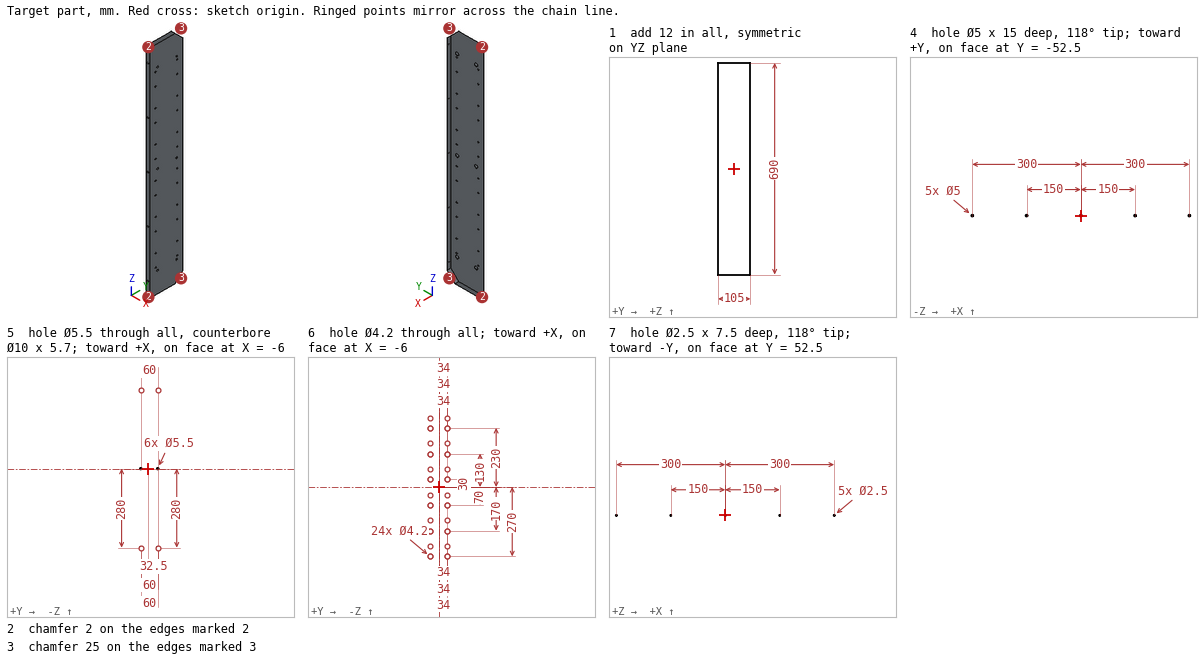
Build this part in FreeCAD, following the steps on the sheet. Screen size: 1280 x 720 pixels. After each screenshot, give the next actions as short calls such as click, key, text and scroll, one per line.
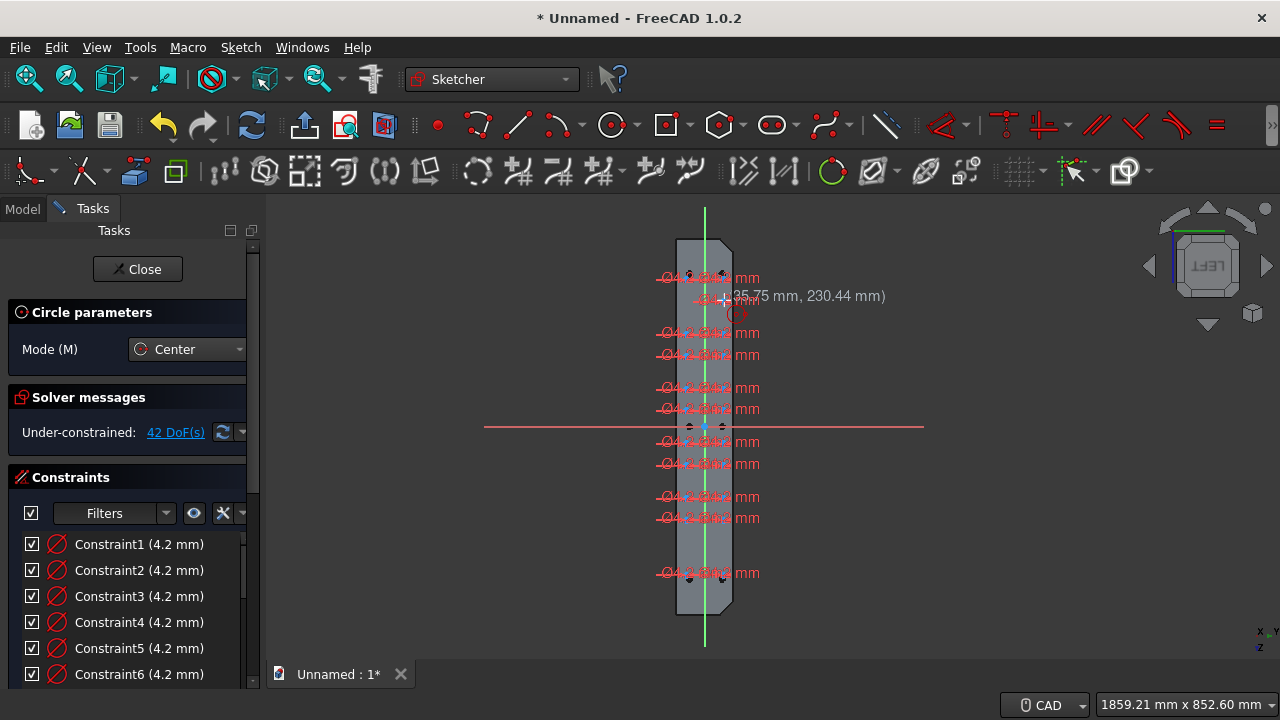
scroll(686, 301, up, 15)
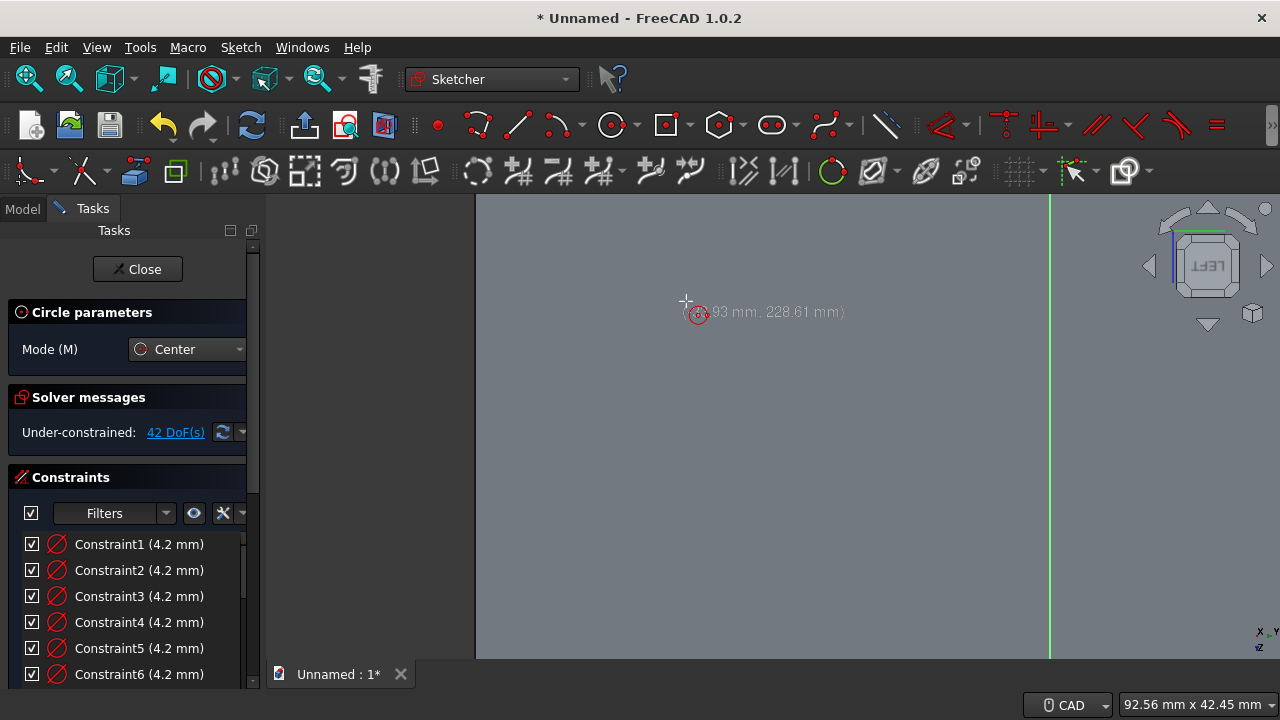
scroll(686, 301, down, 15)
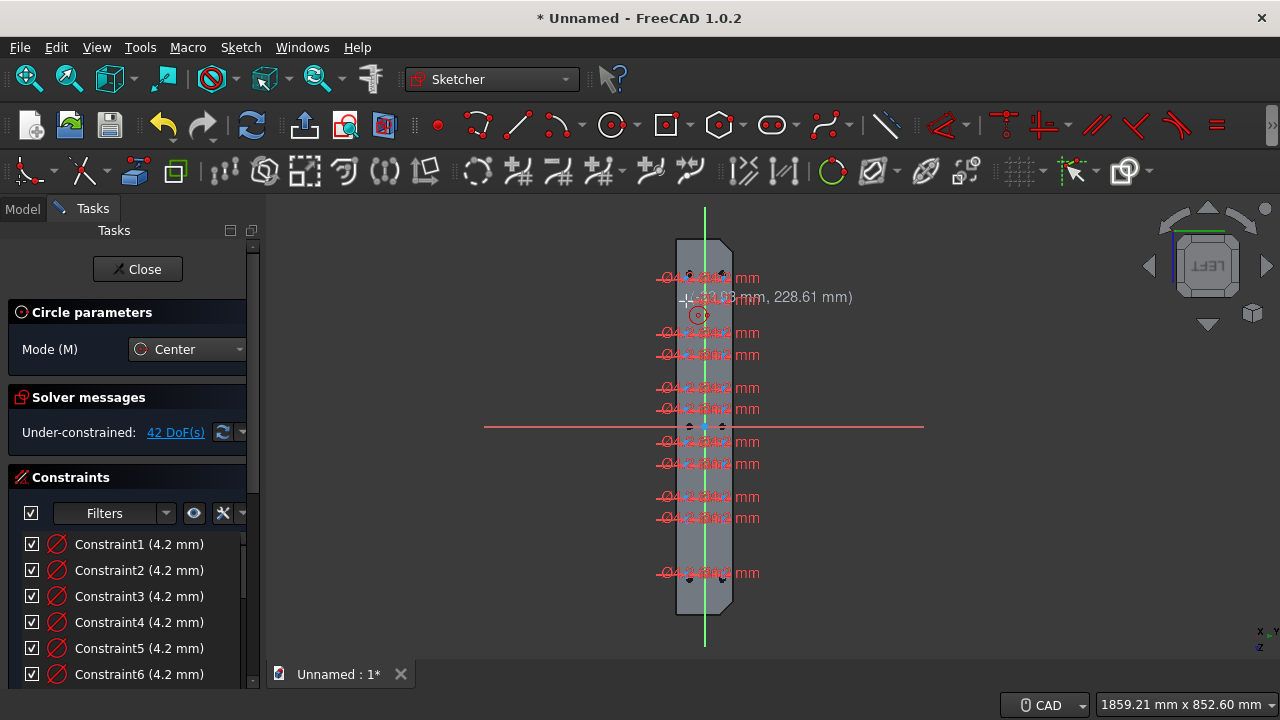
click(686, 301)
move(687, 300)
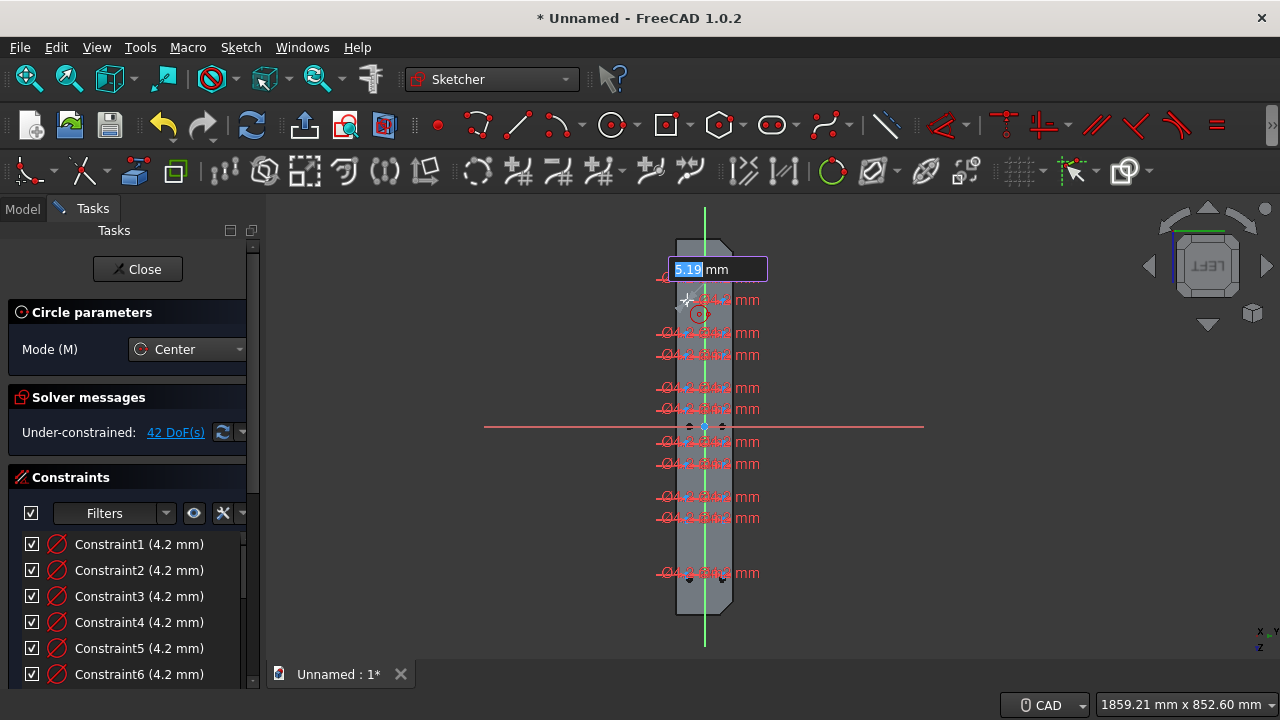
text(4.2)
key(Return)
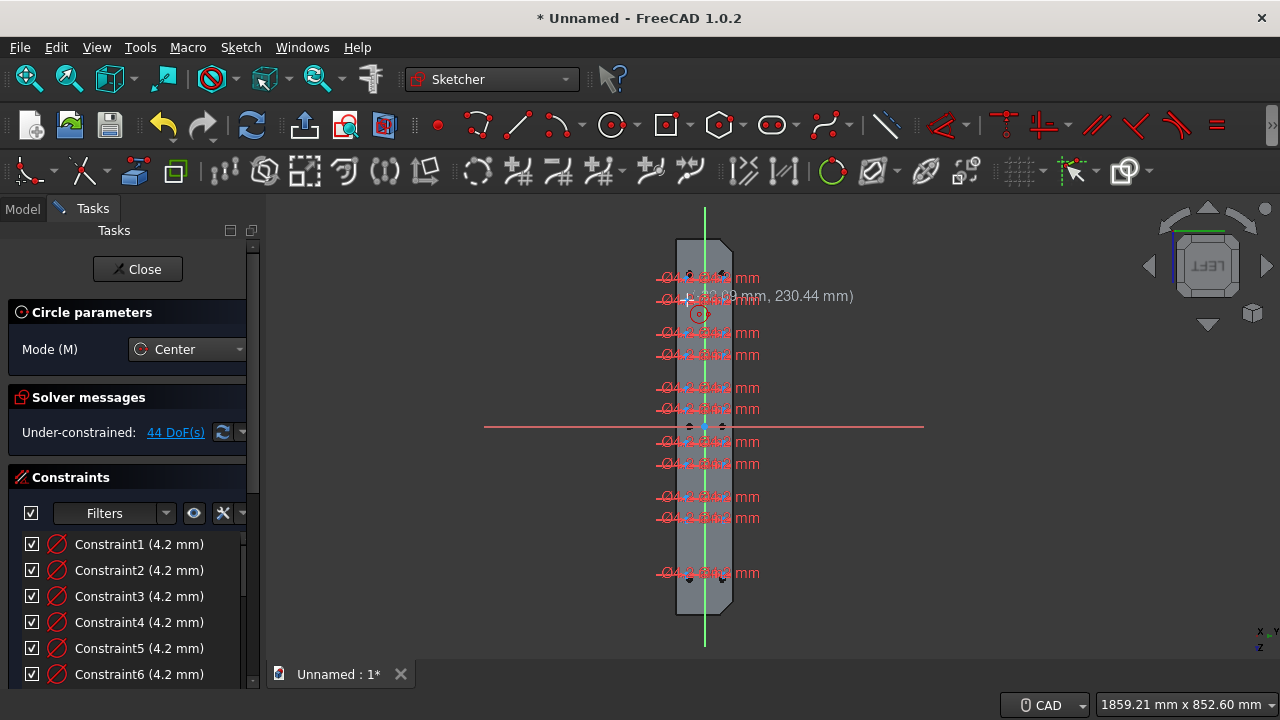
scroll(686, 552, up, 15)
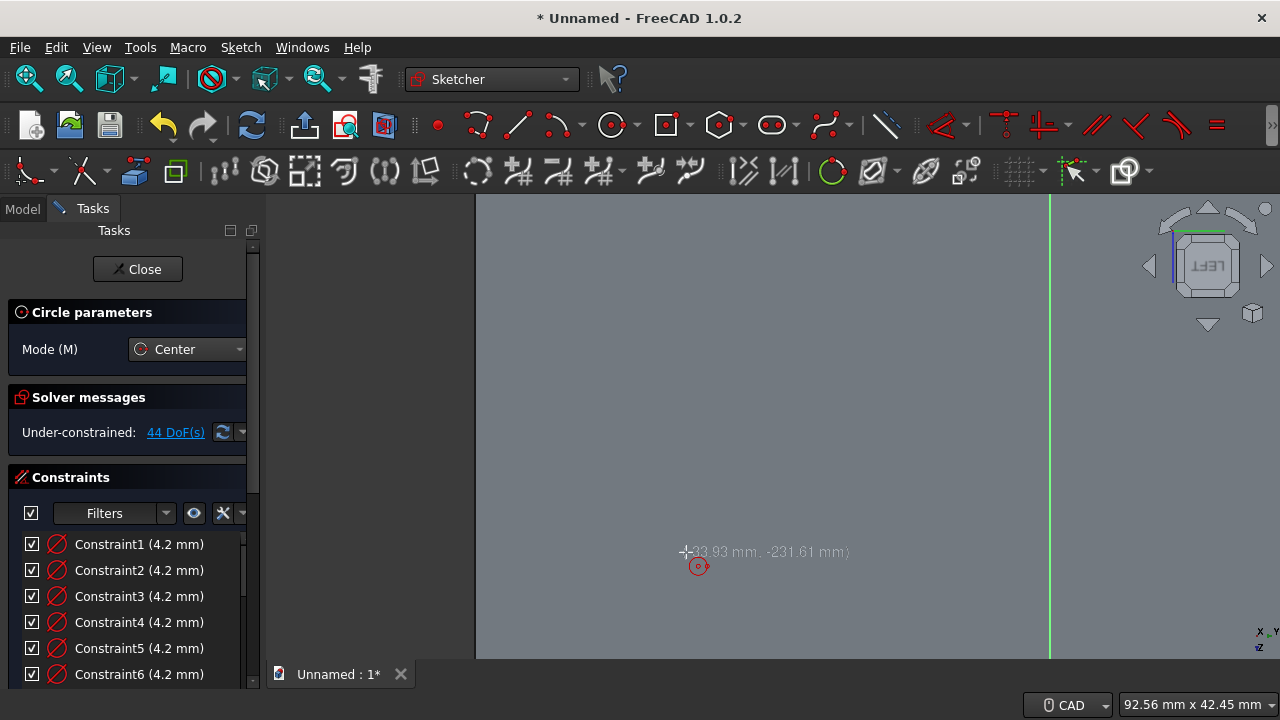
scroll(686, 553, down, 15)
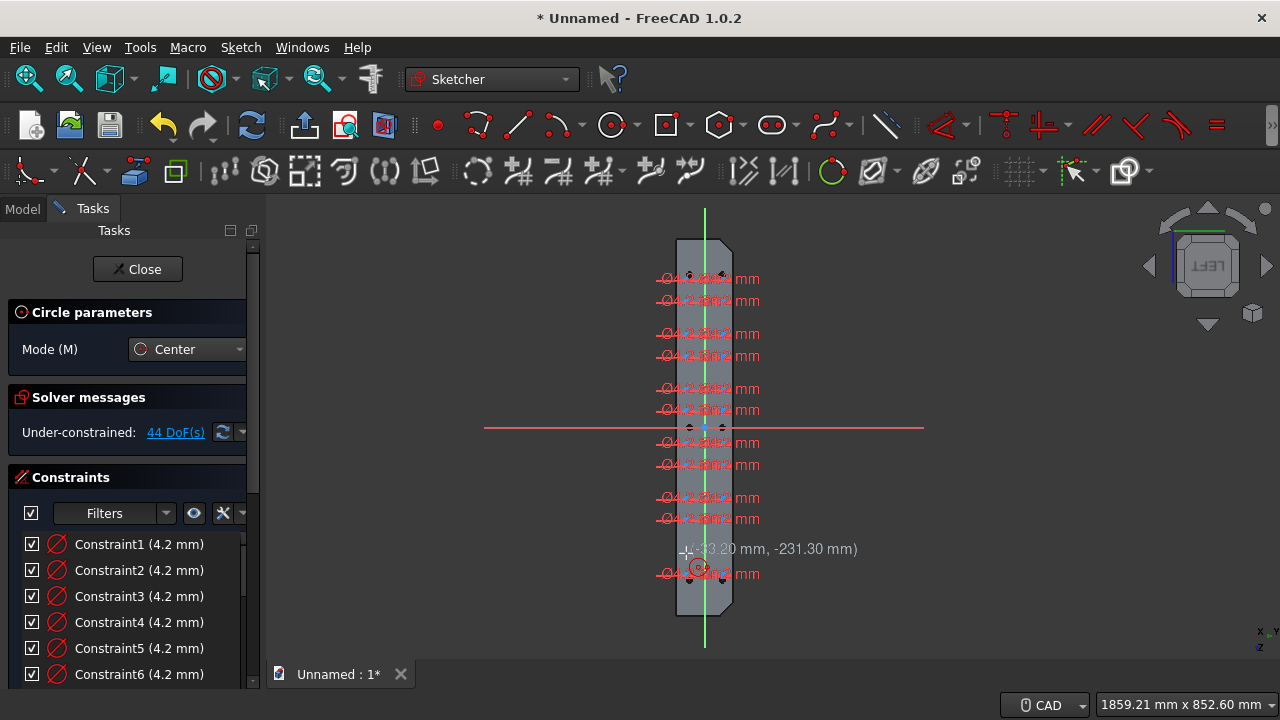
click(686, 553)
move(687, 552)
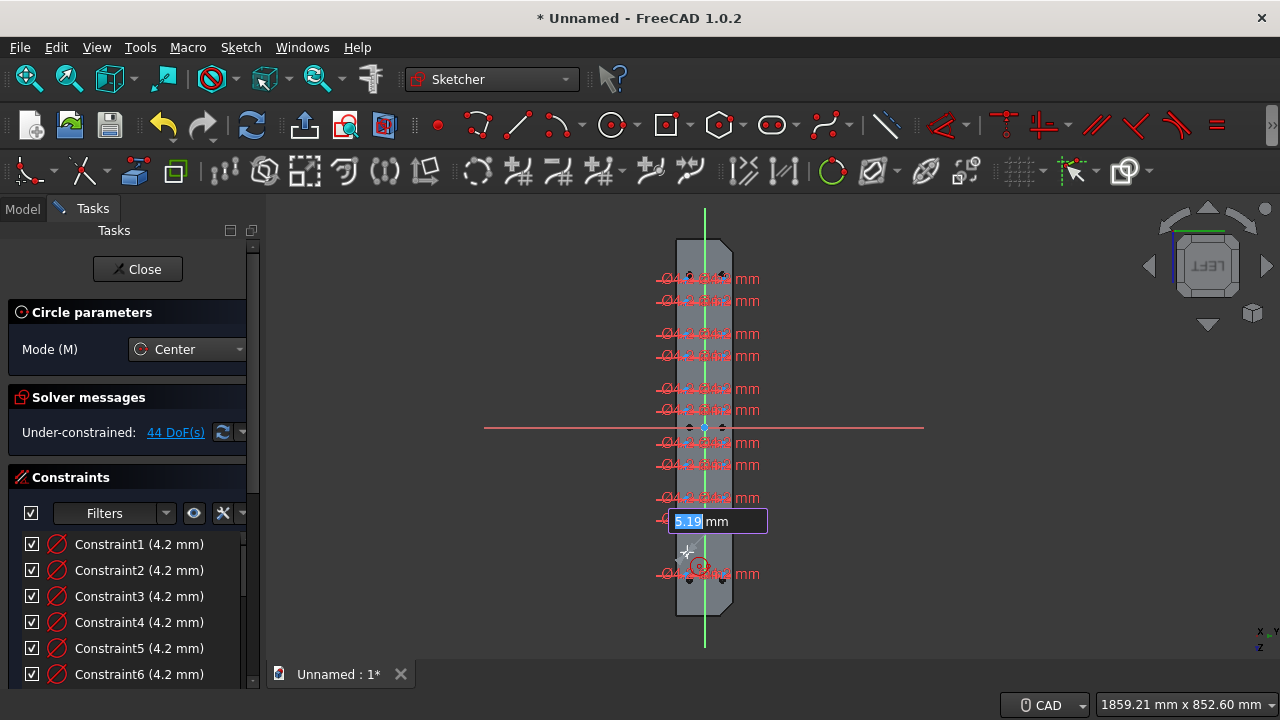
text(4.2)
key(Return)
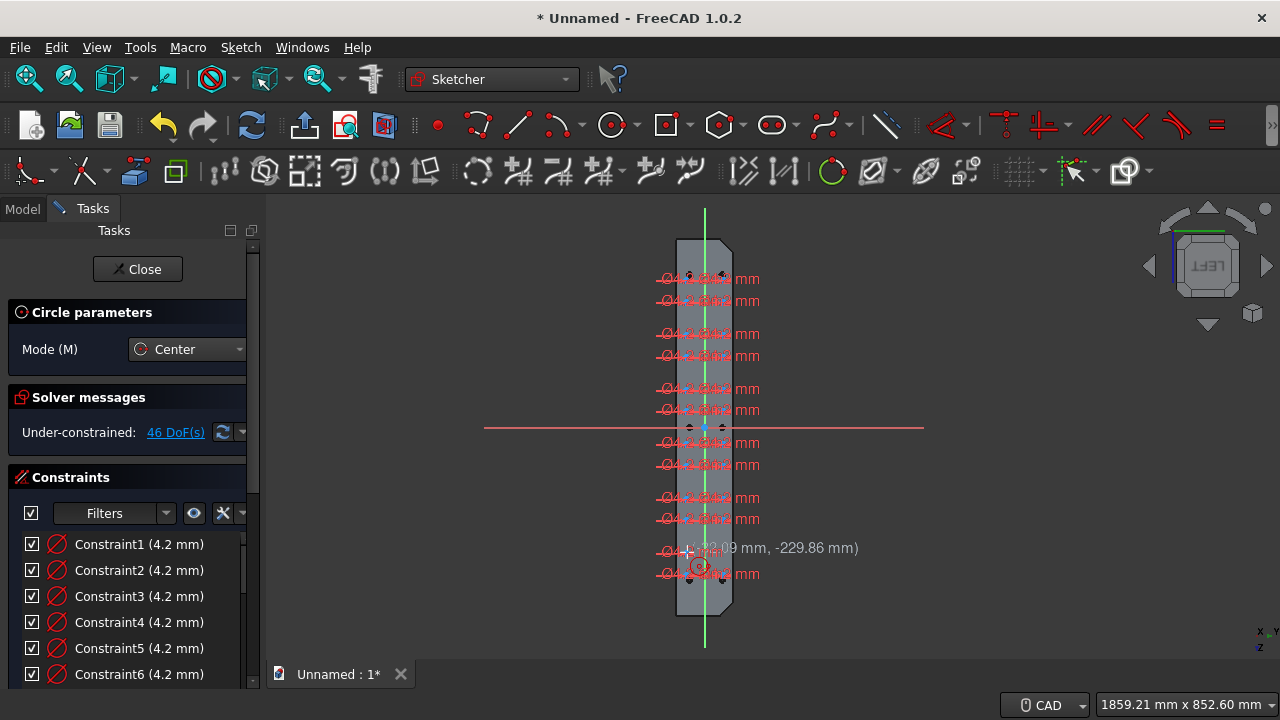
scroll(723, 553, up, 15)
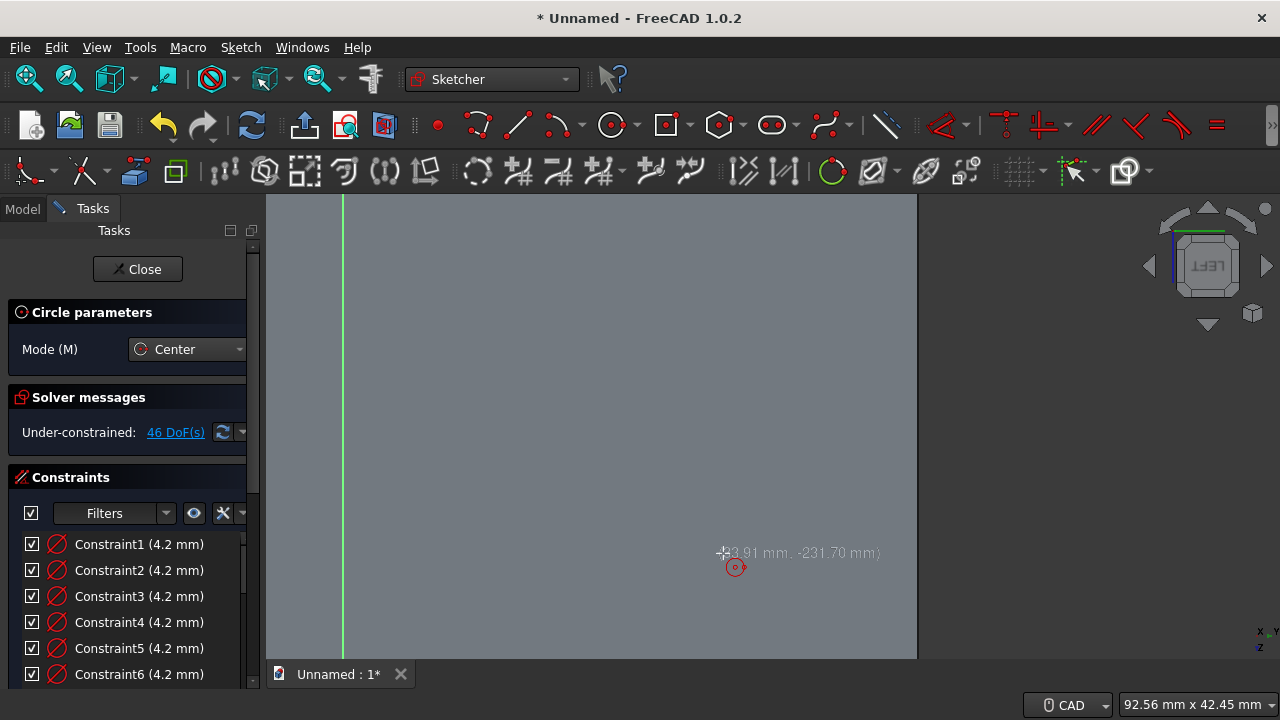
scroll(723, 553, down, 15)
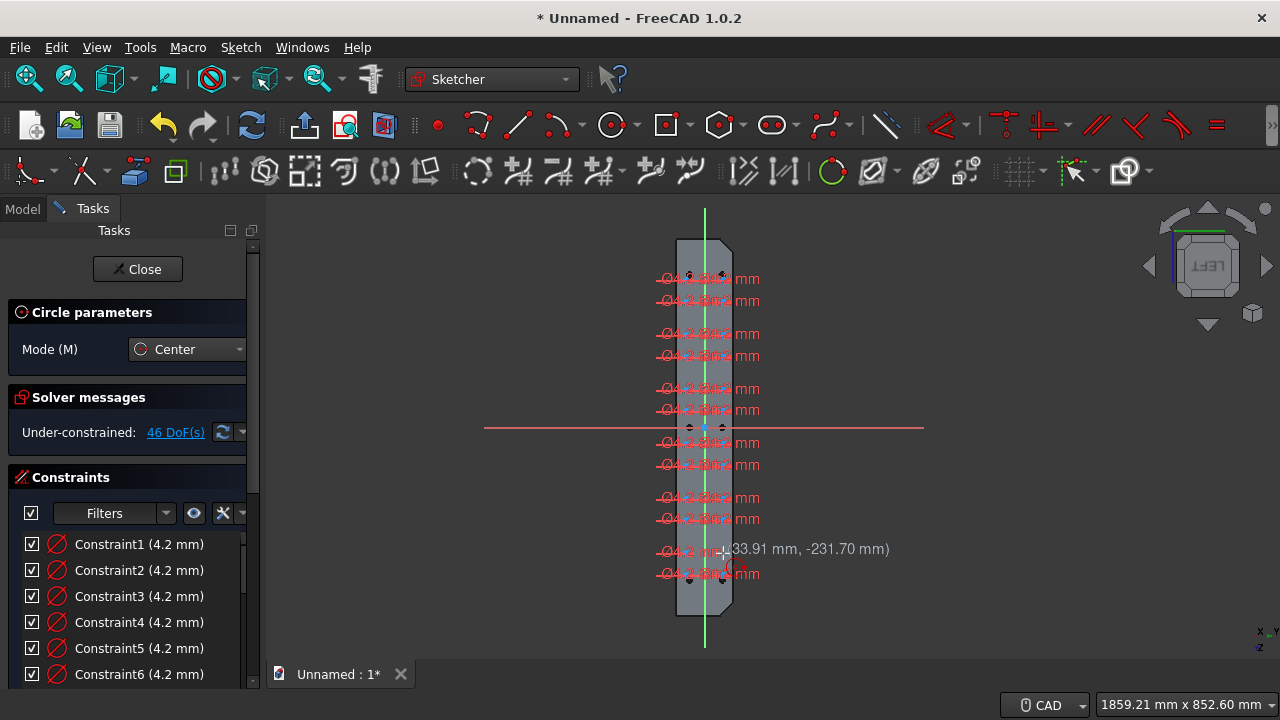
click(723, 553)
move(724, 552)